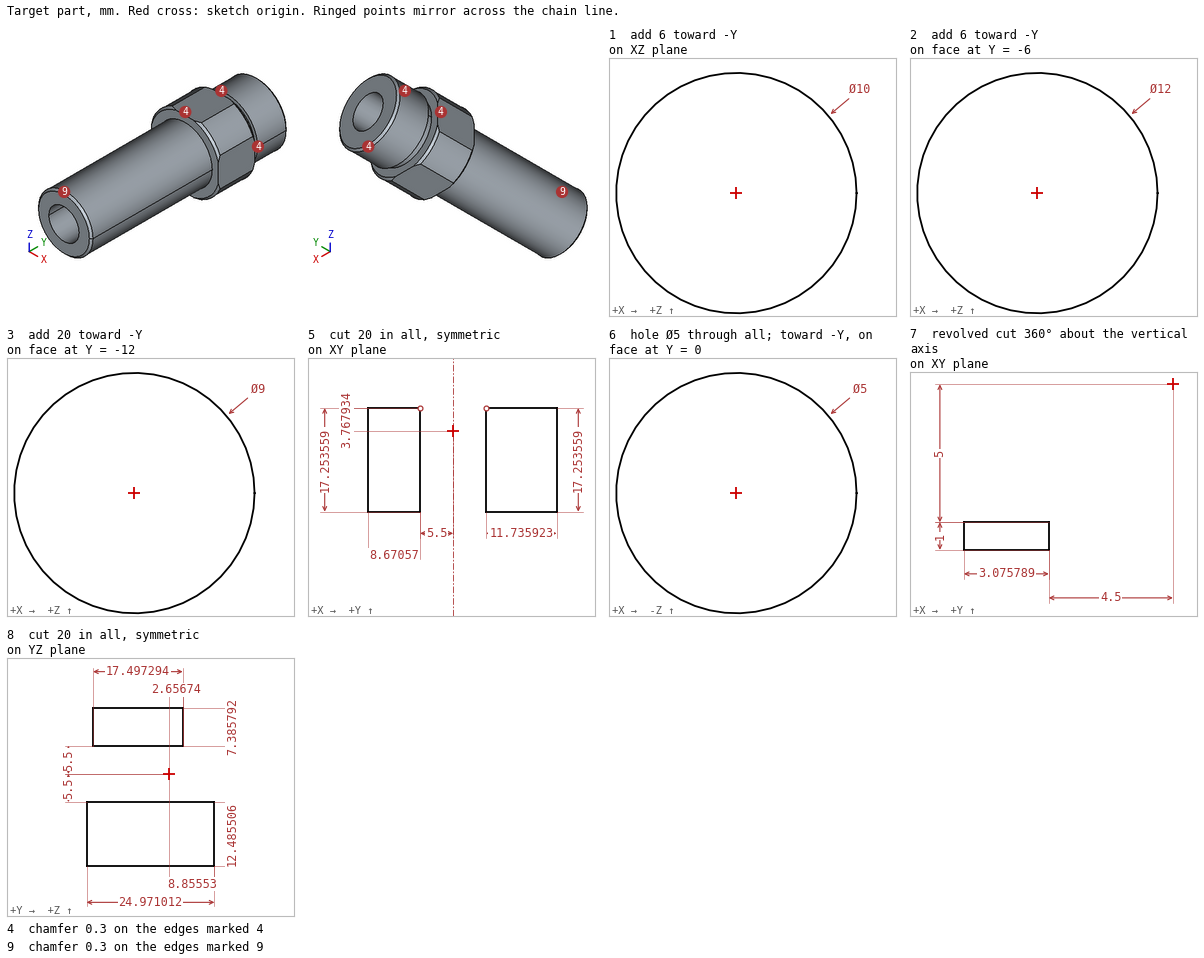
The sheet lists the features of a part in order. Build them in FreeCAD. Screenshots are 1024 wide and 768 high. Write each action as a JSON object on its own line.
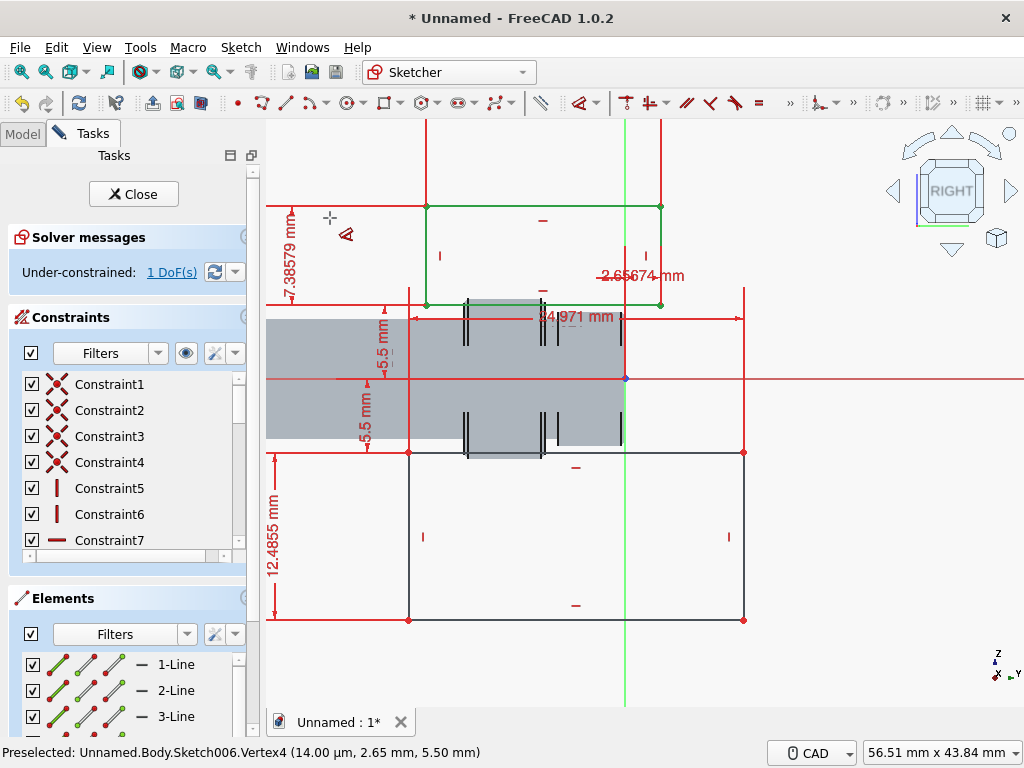
{"action": "left_click", "coordinate": [744, 620]}
{"action": "left_click", "coordinate": [684, 654]}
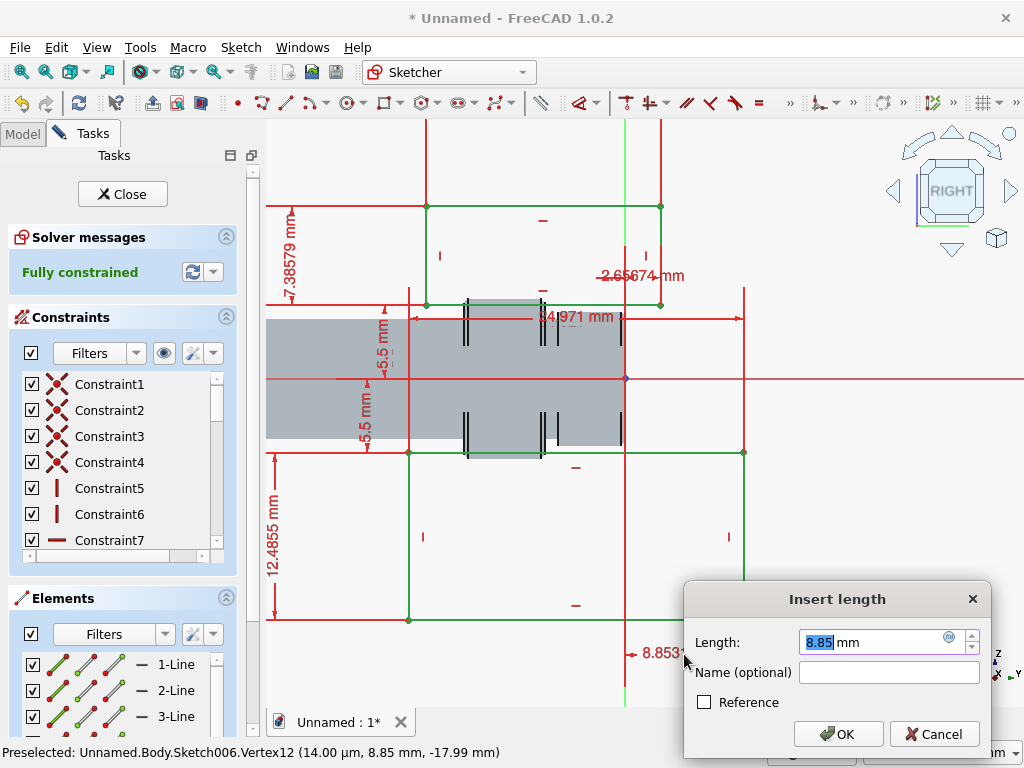
{"action": "type", "text": "8.85553"}
{"action": "key", "text": "Return"}
{"action": "key", "text": "Escape"}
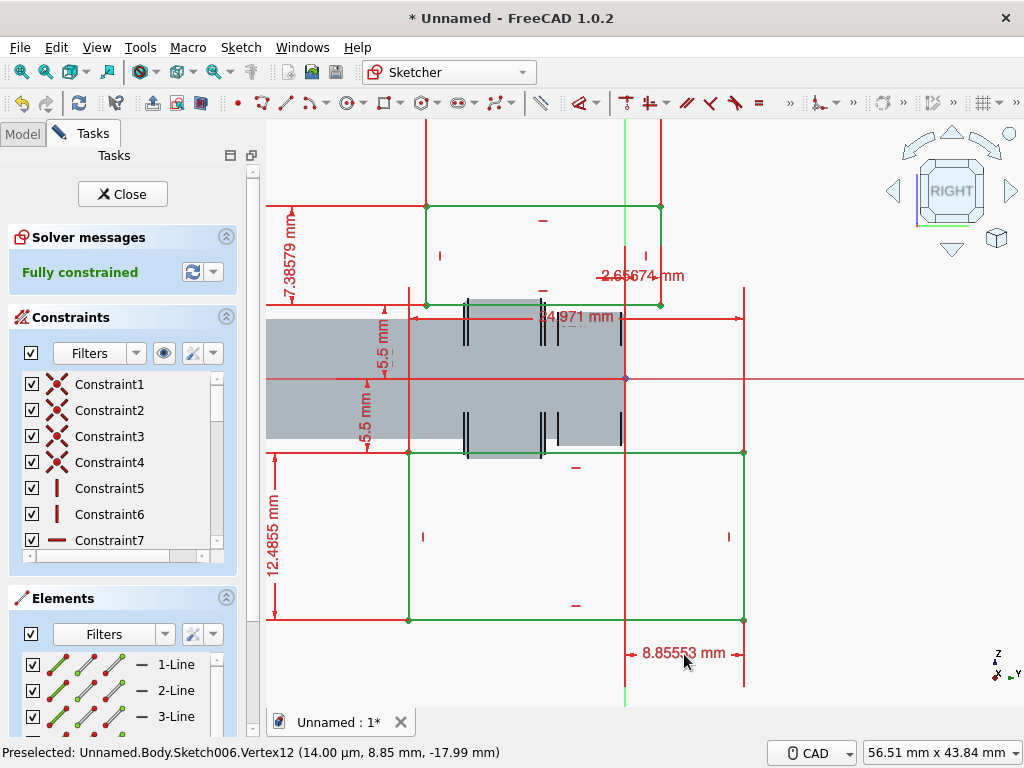
{"action": "left_click", "coordinate": [123, 194]}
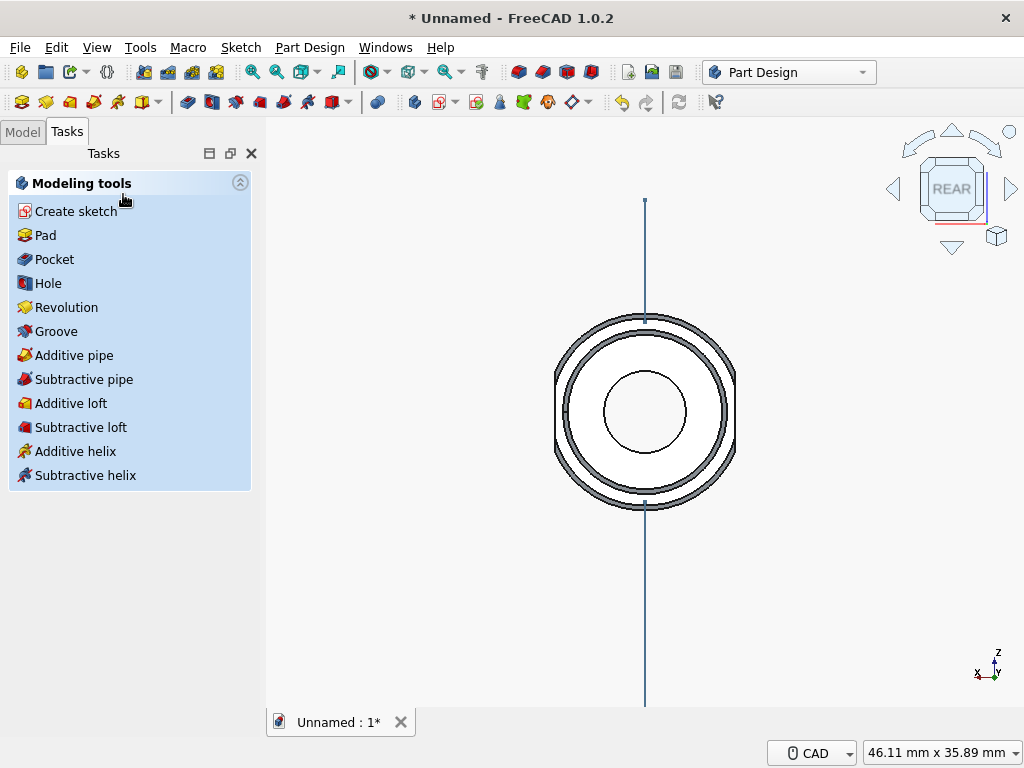
{"action": "left_click", "coordinate": [188, 102]}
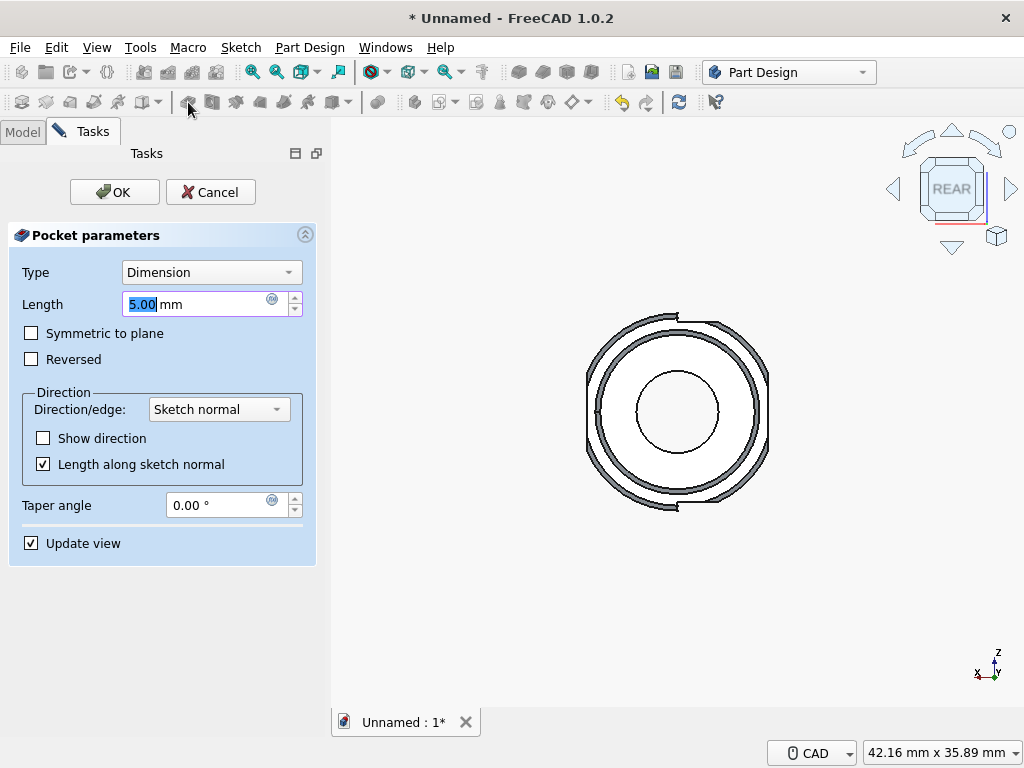
{"action": "type", "text": "20"}
{"action": "key", "text": "Tab"}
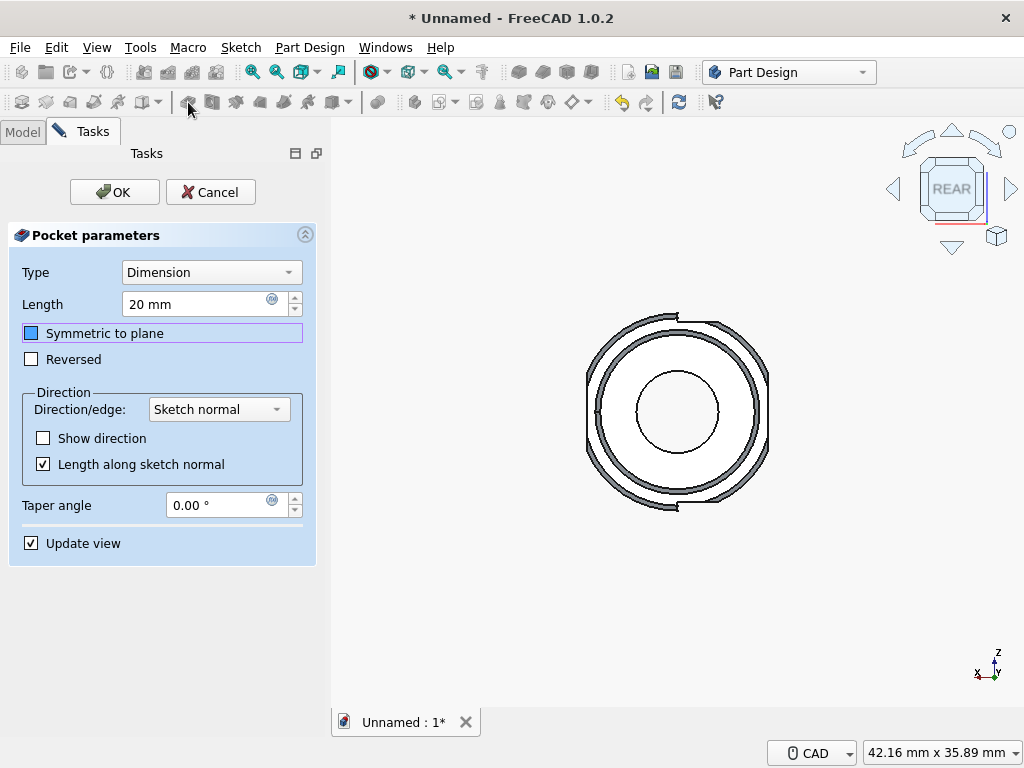
{"action": "left_click", "coordinate": [30, 333]}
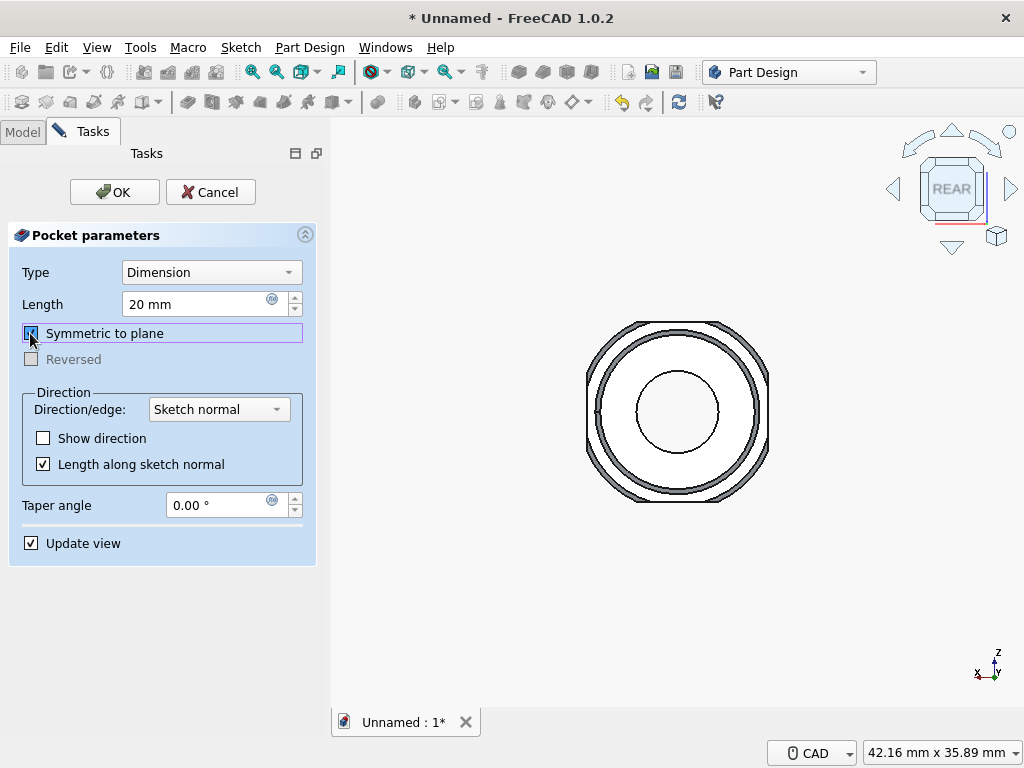
{"action": "left_click", "coordinate": [115, 192]}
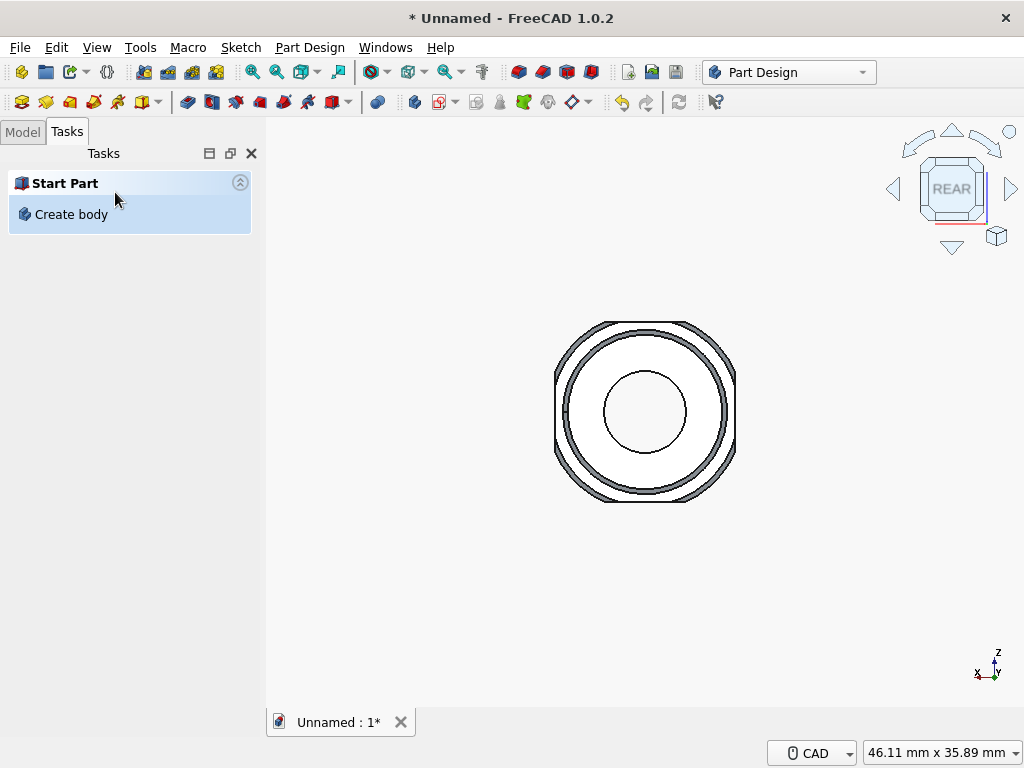
{"action": "key", "text": "v f"}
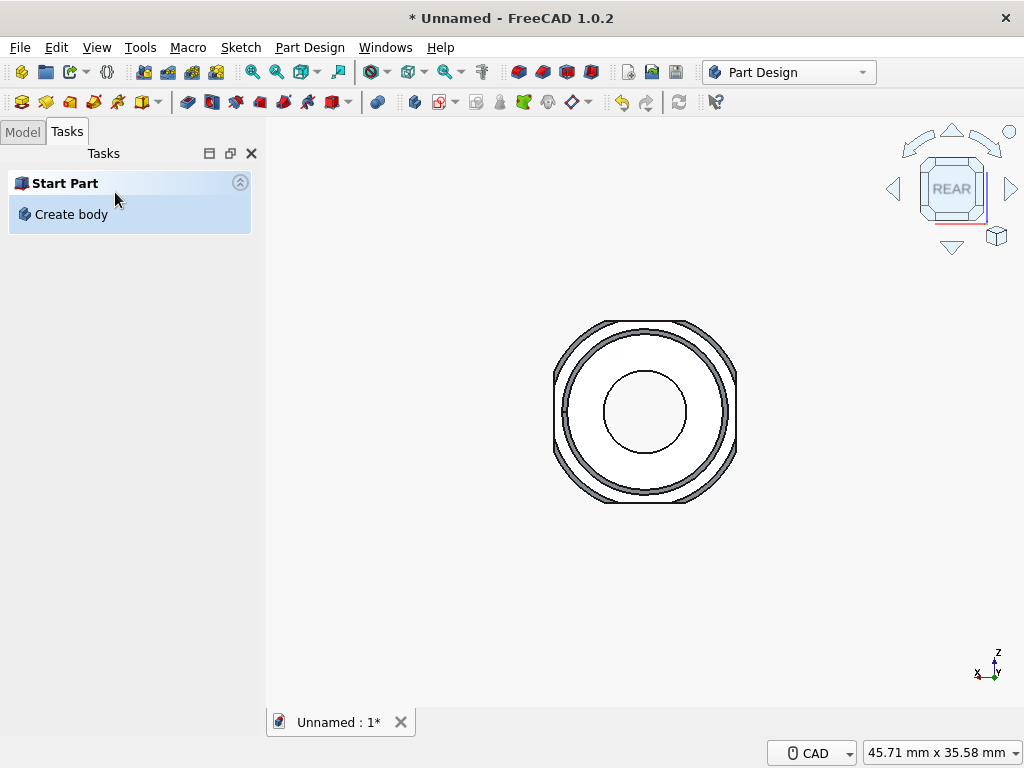
{"action": "key", "text": "0"}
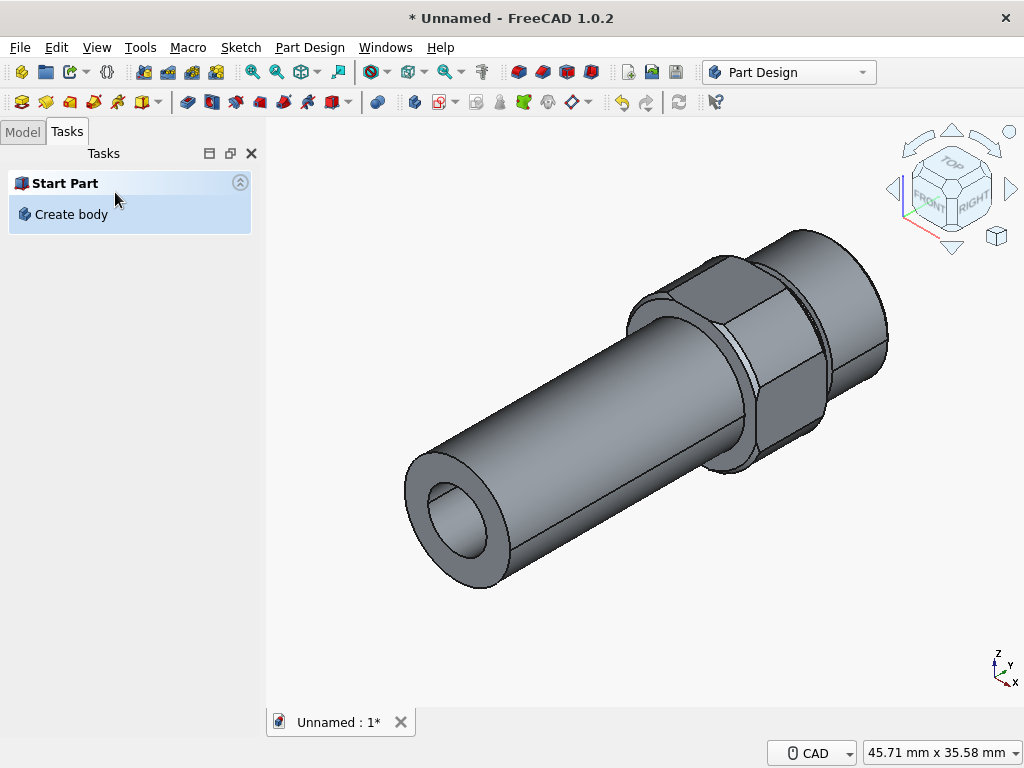
{"action": "left_click", "coordinate": [441, 452]}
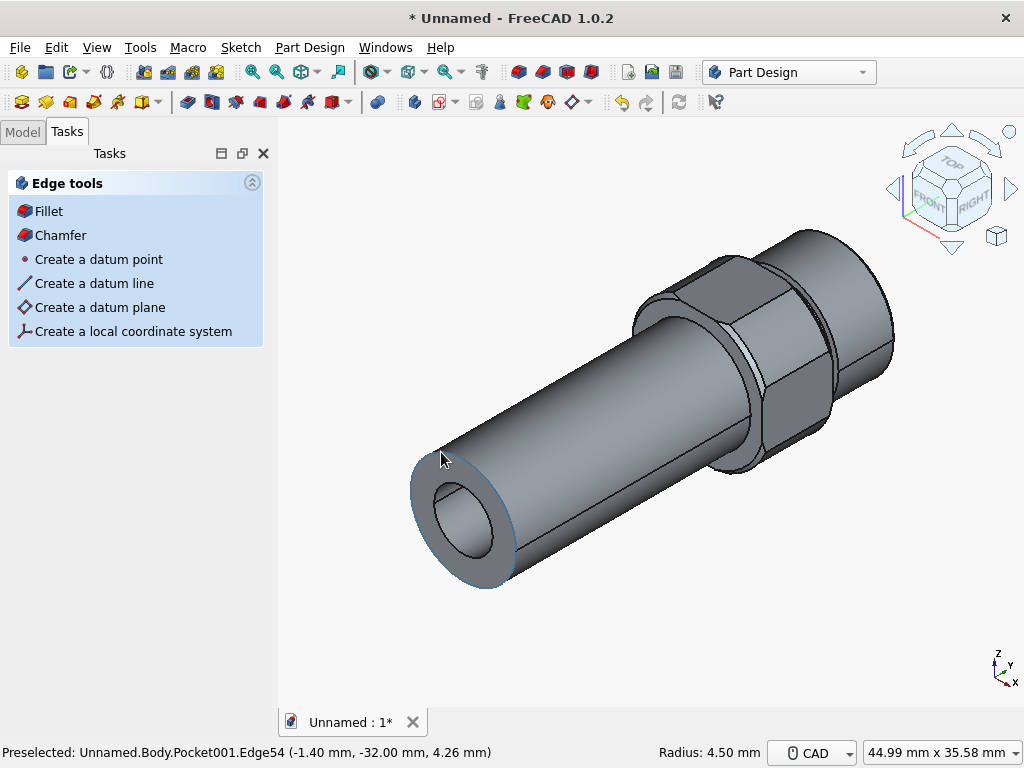
{"action": "left_click", "coordinate": [544, 72]}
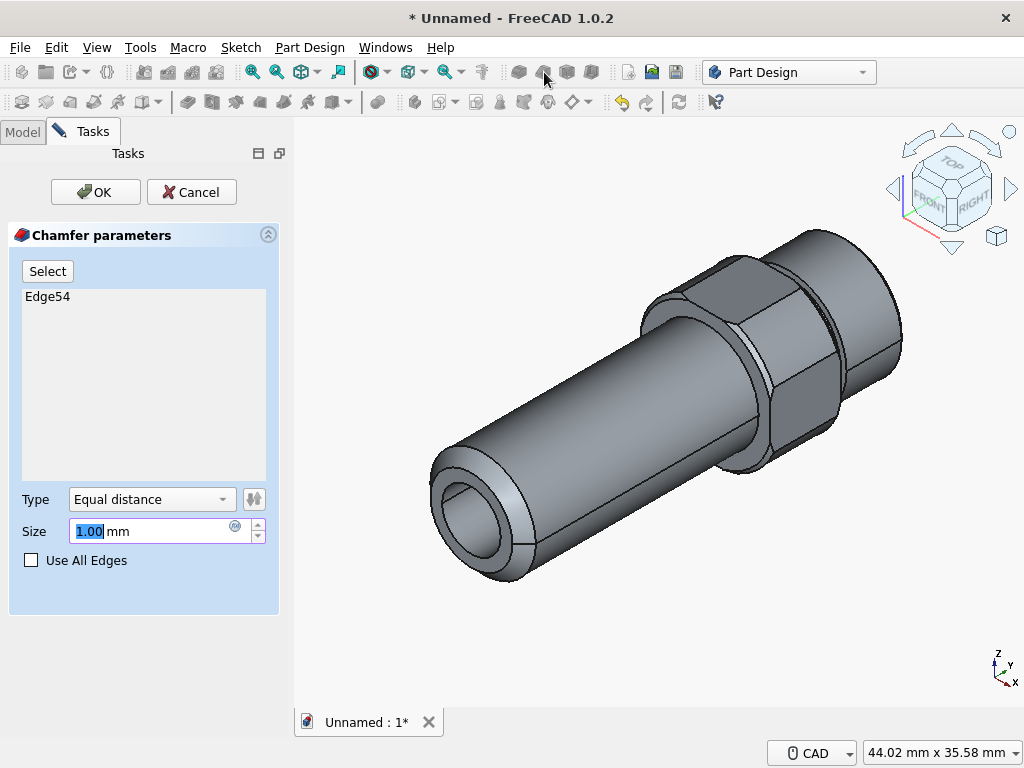
{"action": "type", "text": "0.3"}
{"action": "key", "text": "Tab"}